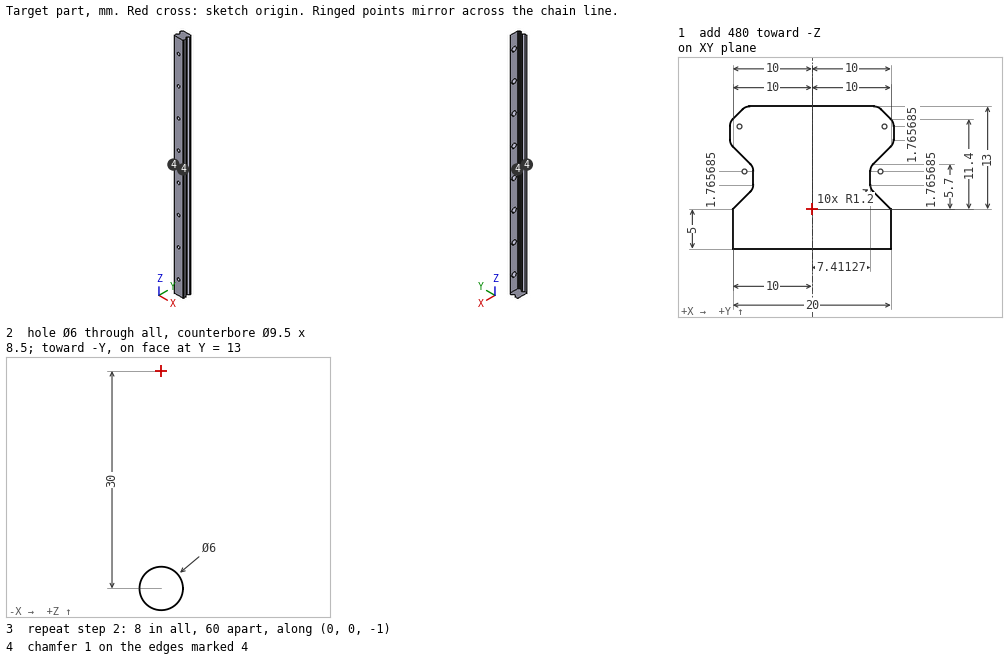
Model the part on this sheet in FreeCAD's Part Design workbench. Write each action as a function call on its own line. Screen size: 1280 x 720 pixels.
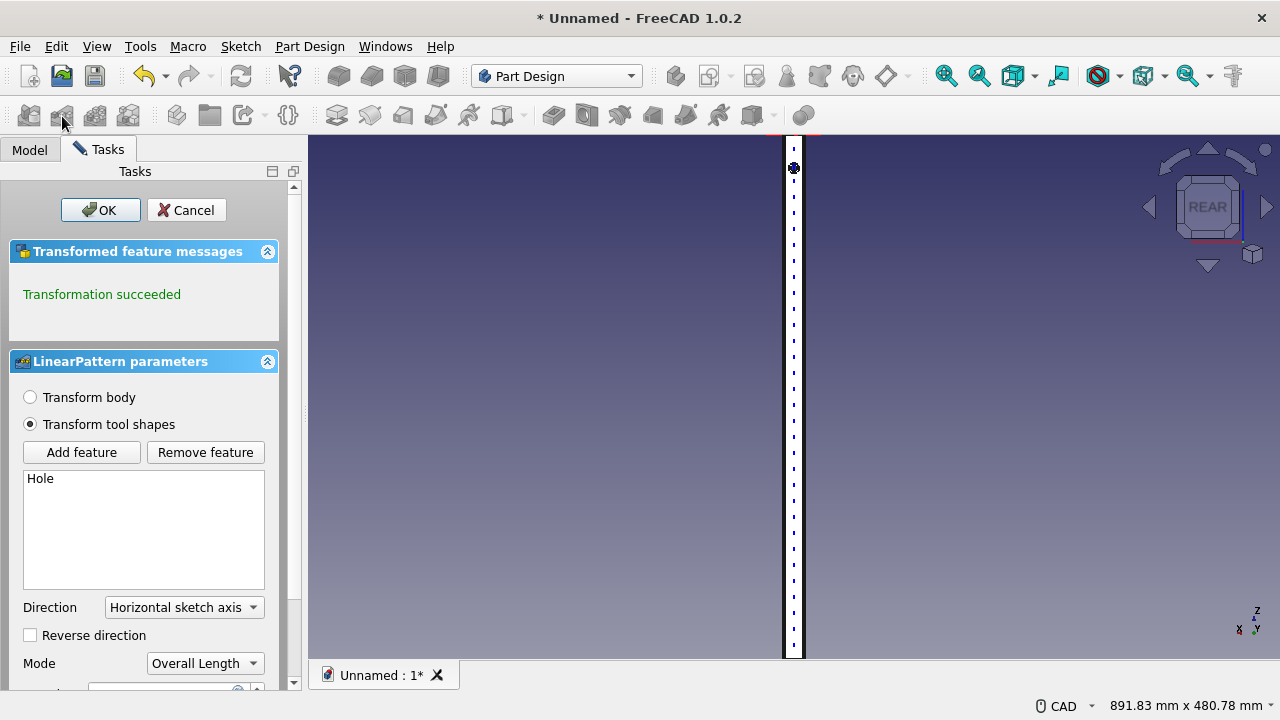
click(185, 608)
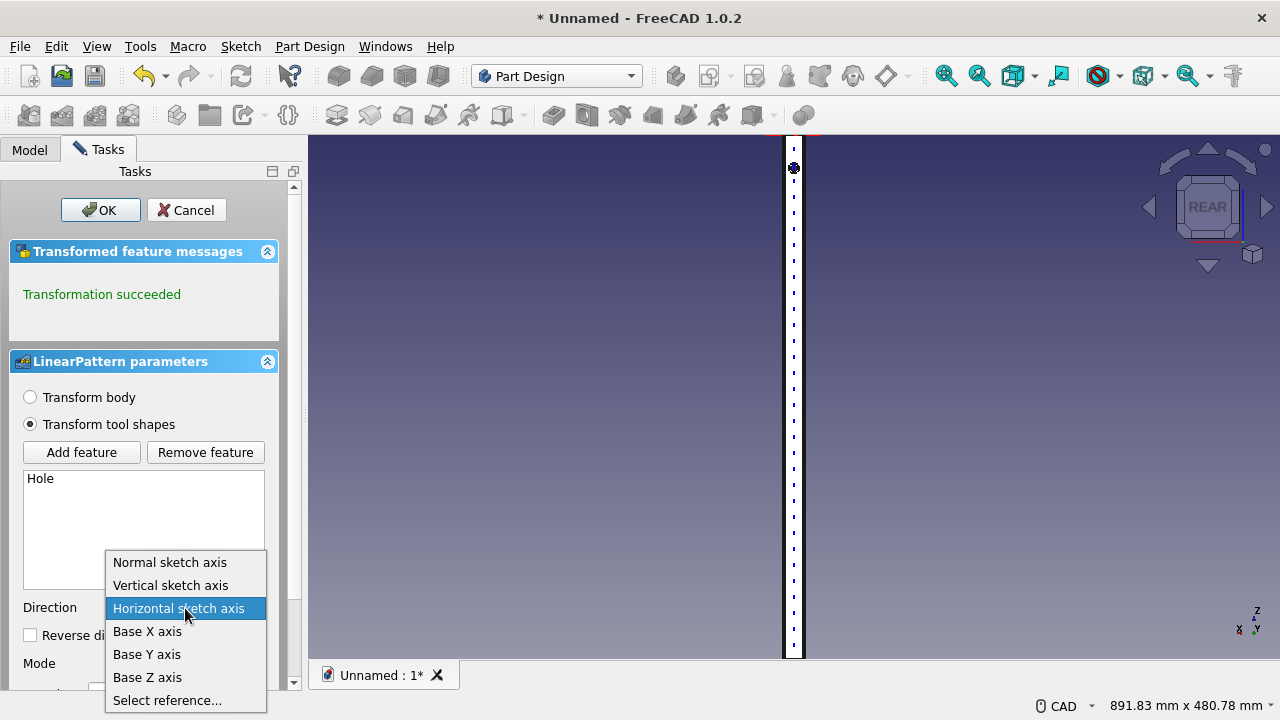
click(184, 678)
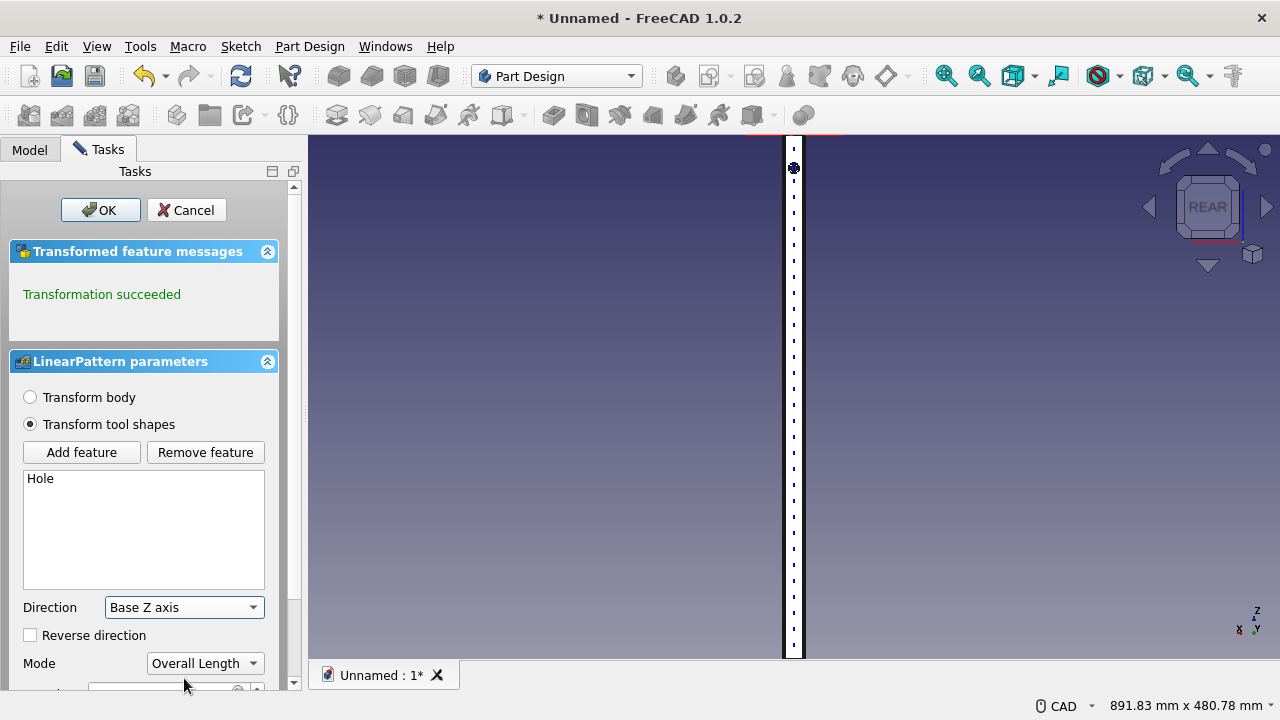
click(206, 664)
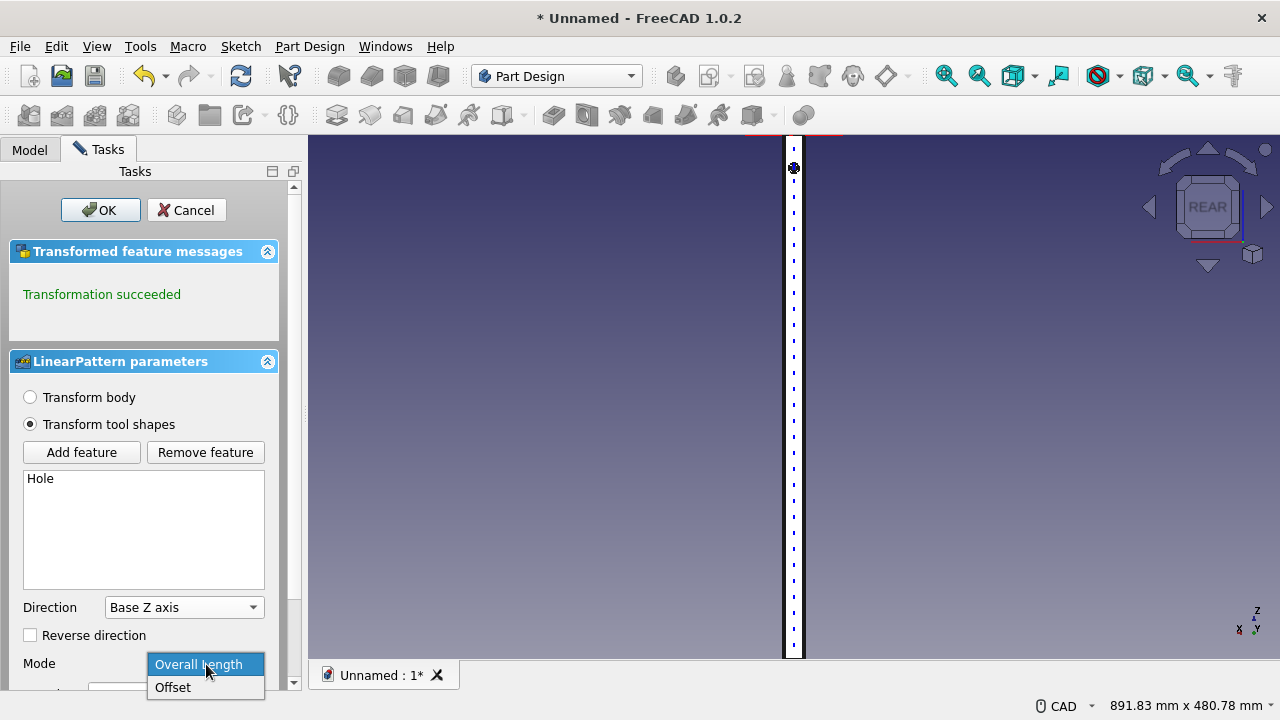
click(204, 688)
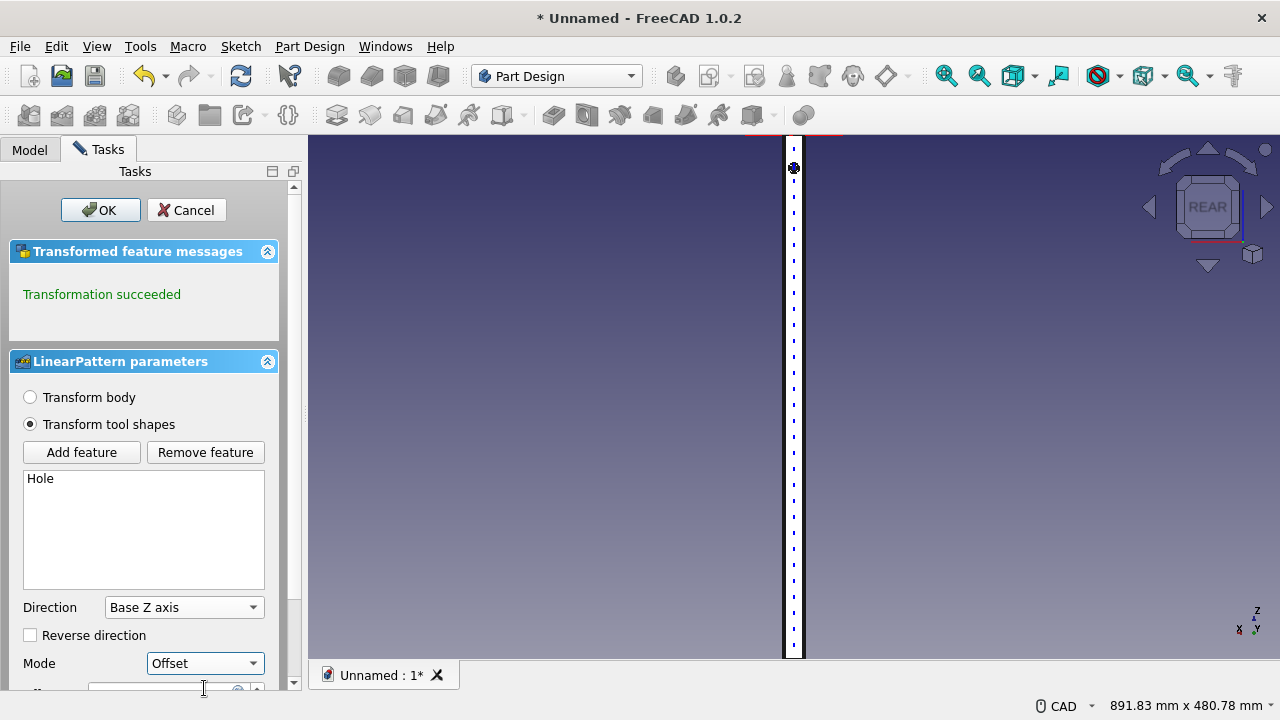
scroll(294, 436, down, 2)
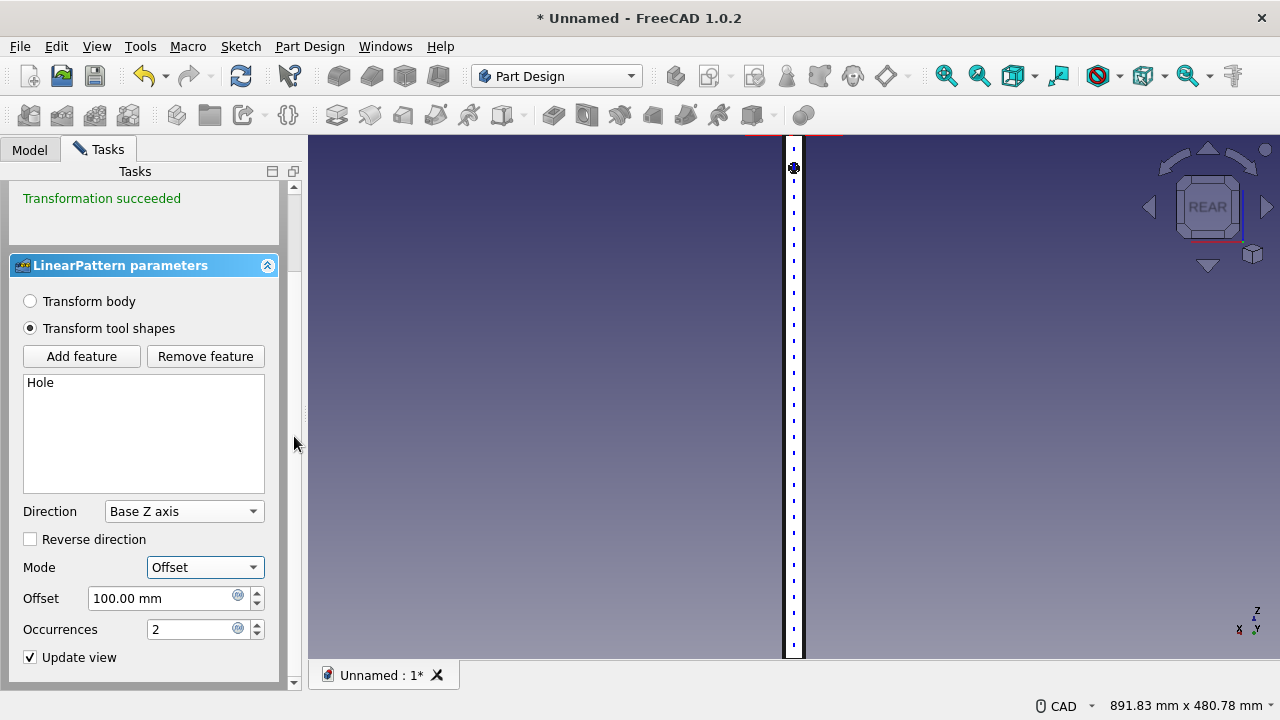
triple_click(170, 598)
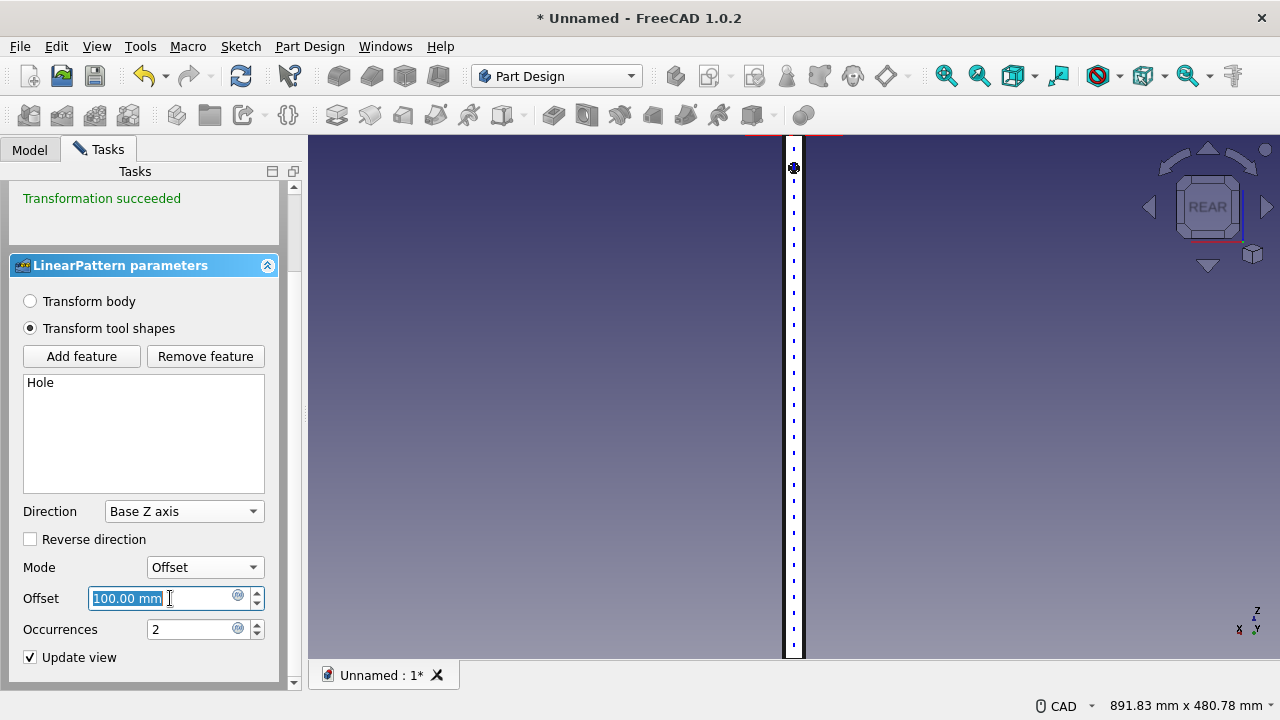
text(60)
key(Tab)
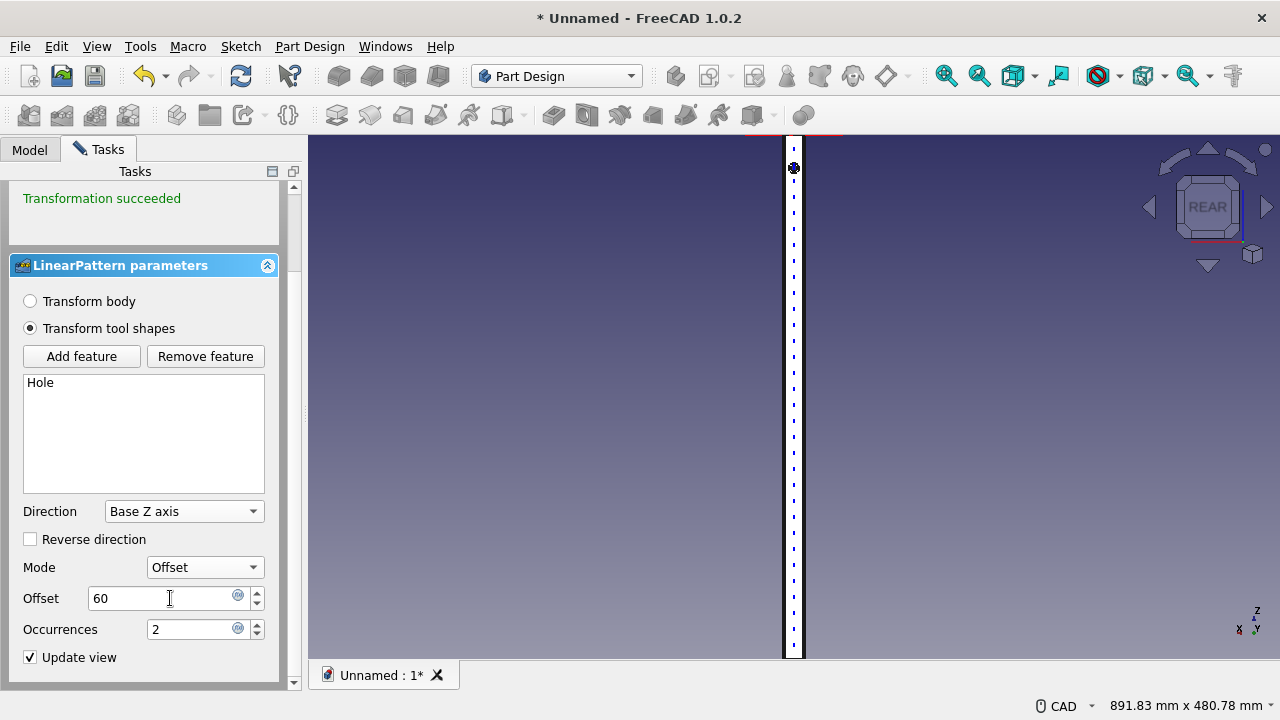
triple_click(199, 630)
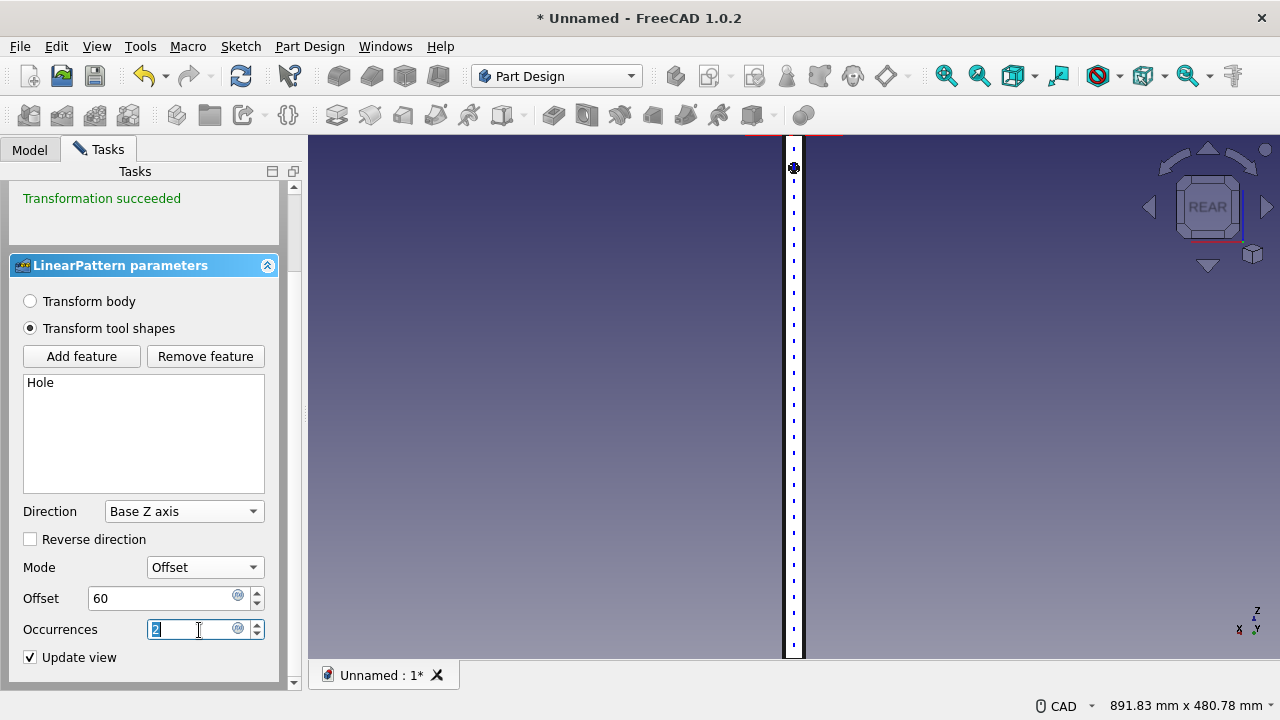
text(8)
key(Tab)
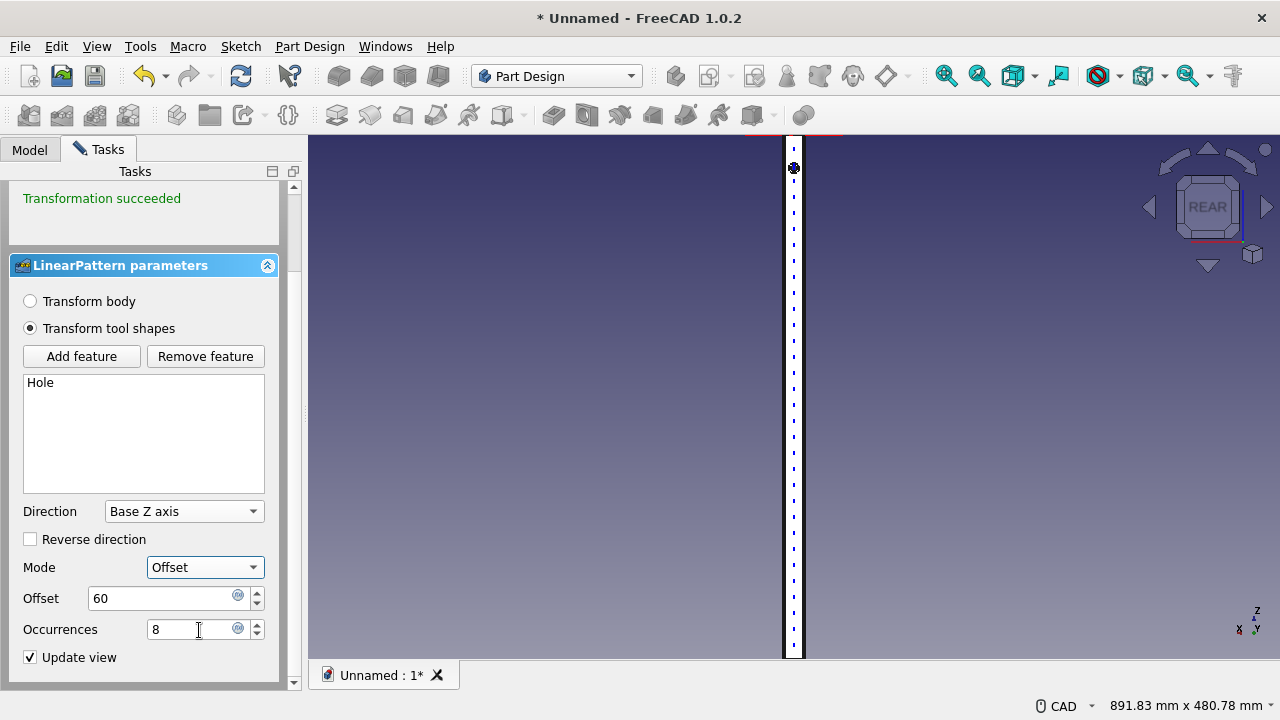
click(31, 539)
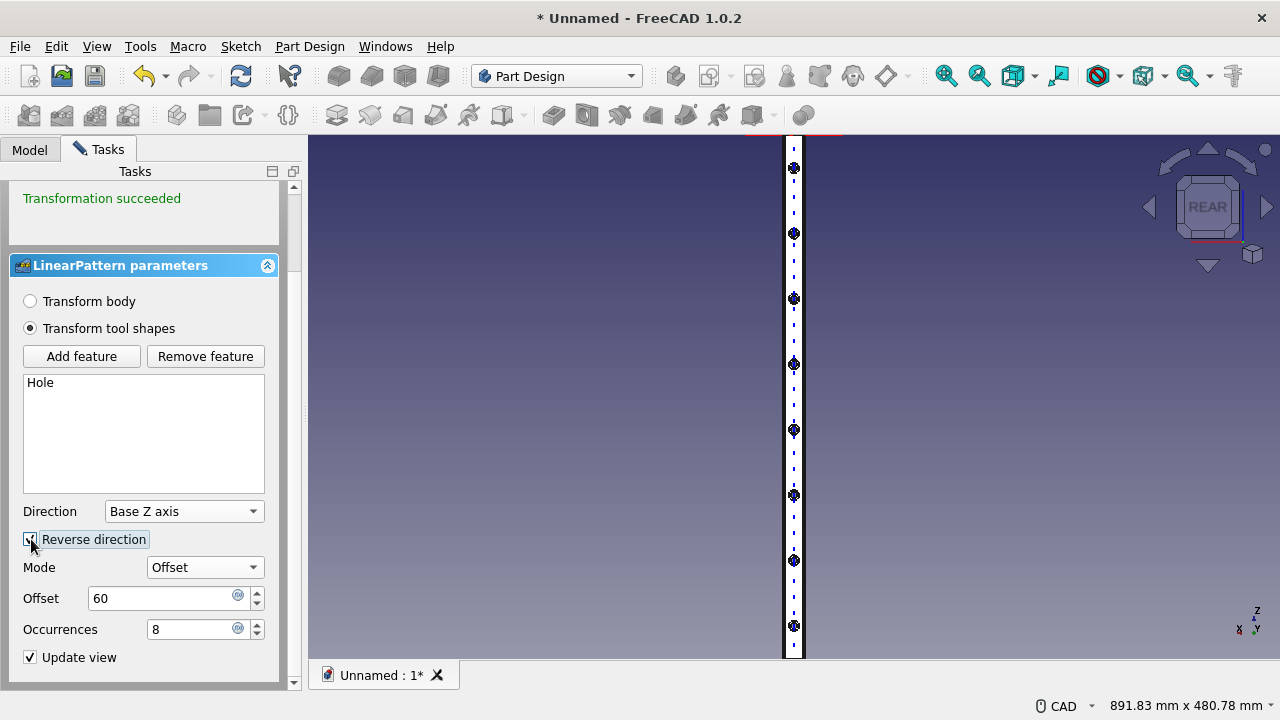
scroll(294, 436, up, 3)